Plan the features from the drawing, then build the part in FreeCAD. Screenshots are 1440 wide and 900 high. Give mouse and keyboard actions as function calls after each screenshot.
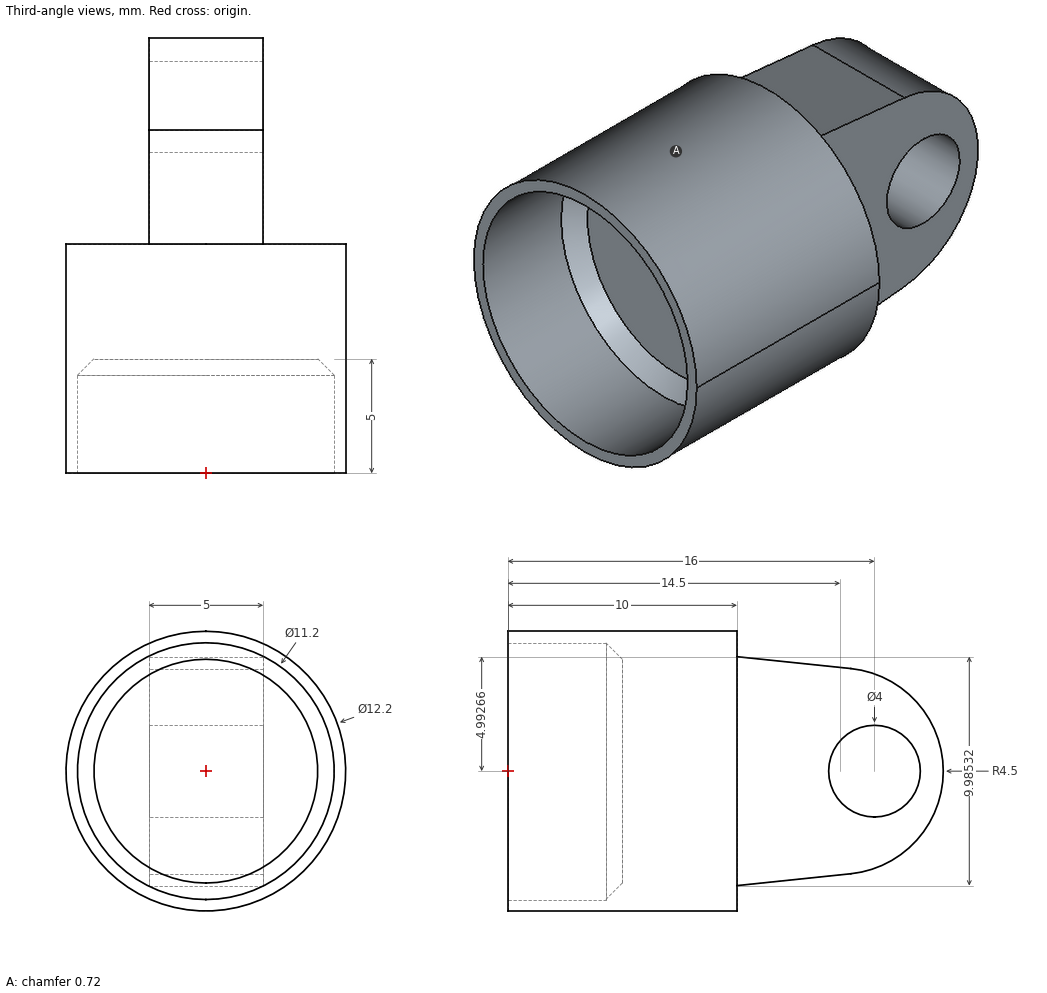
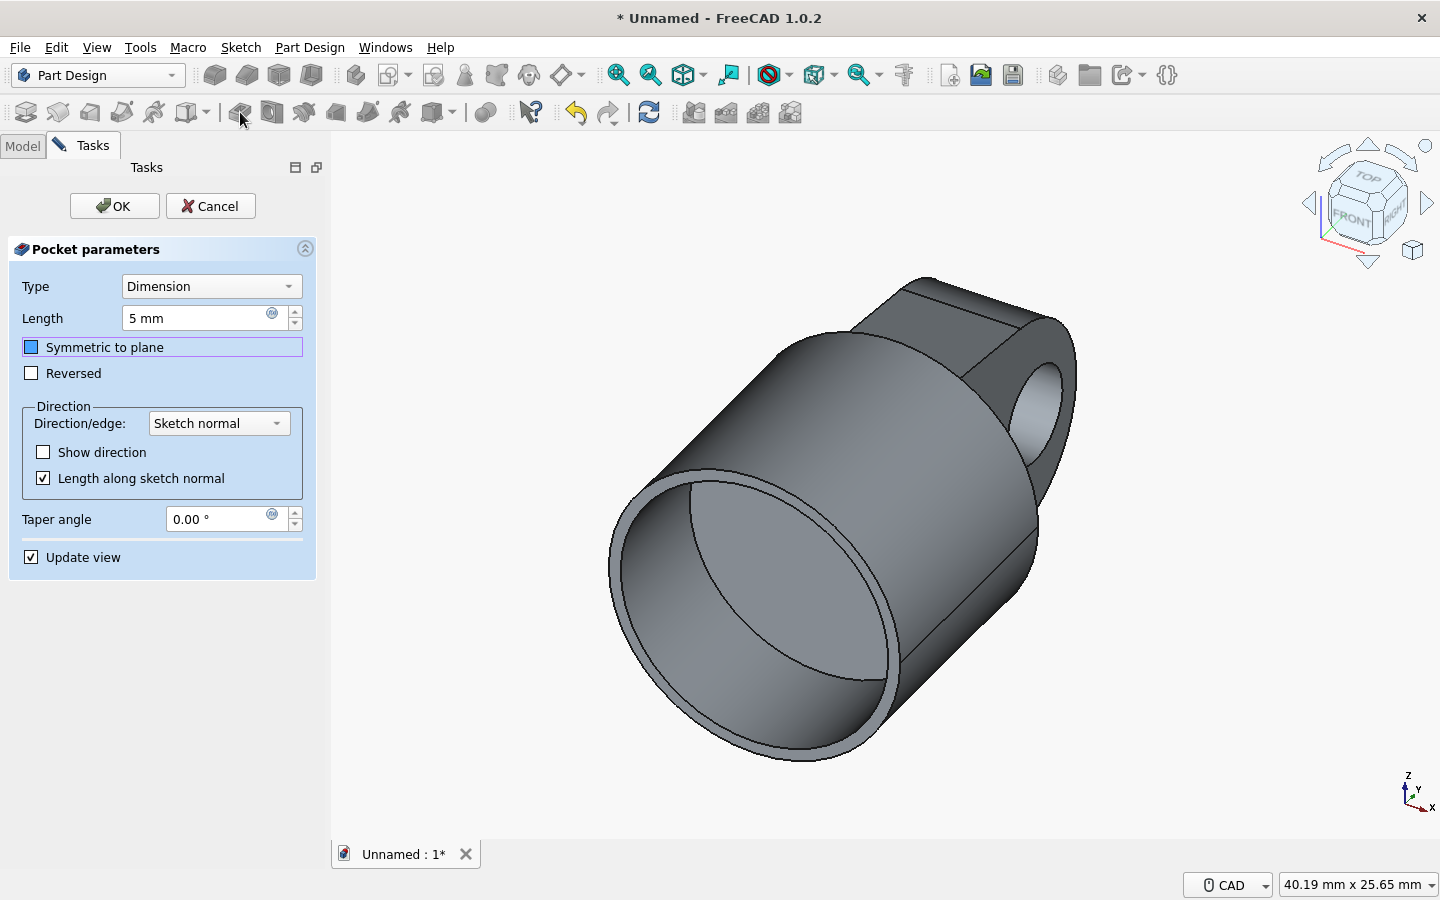
click(115, 206)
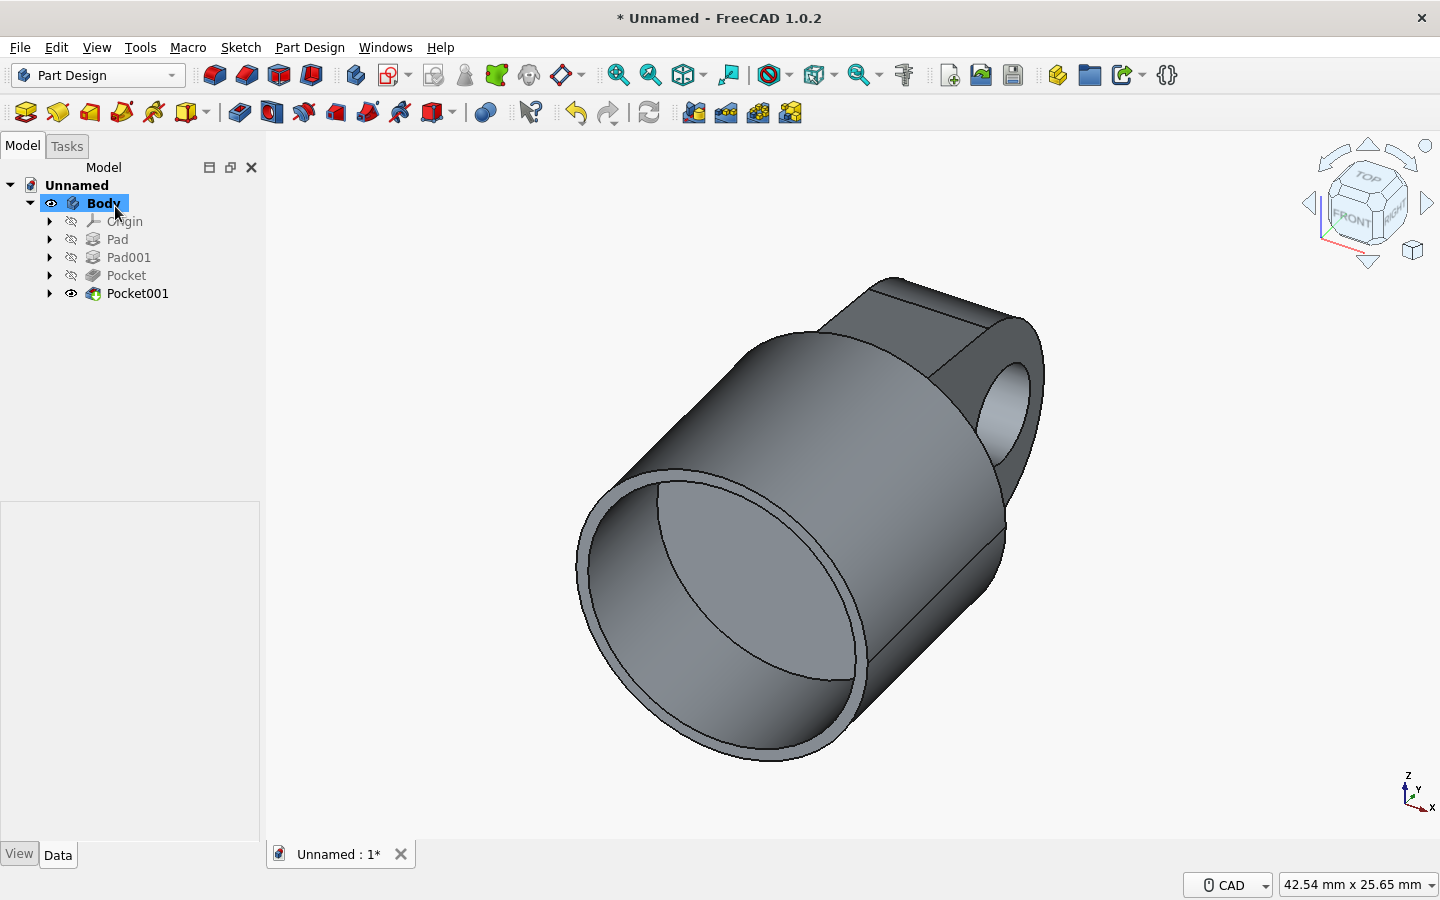
key(0)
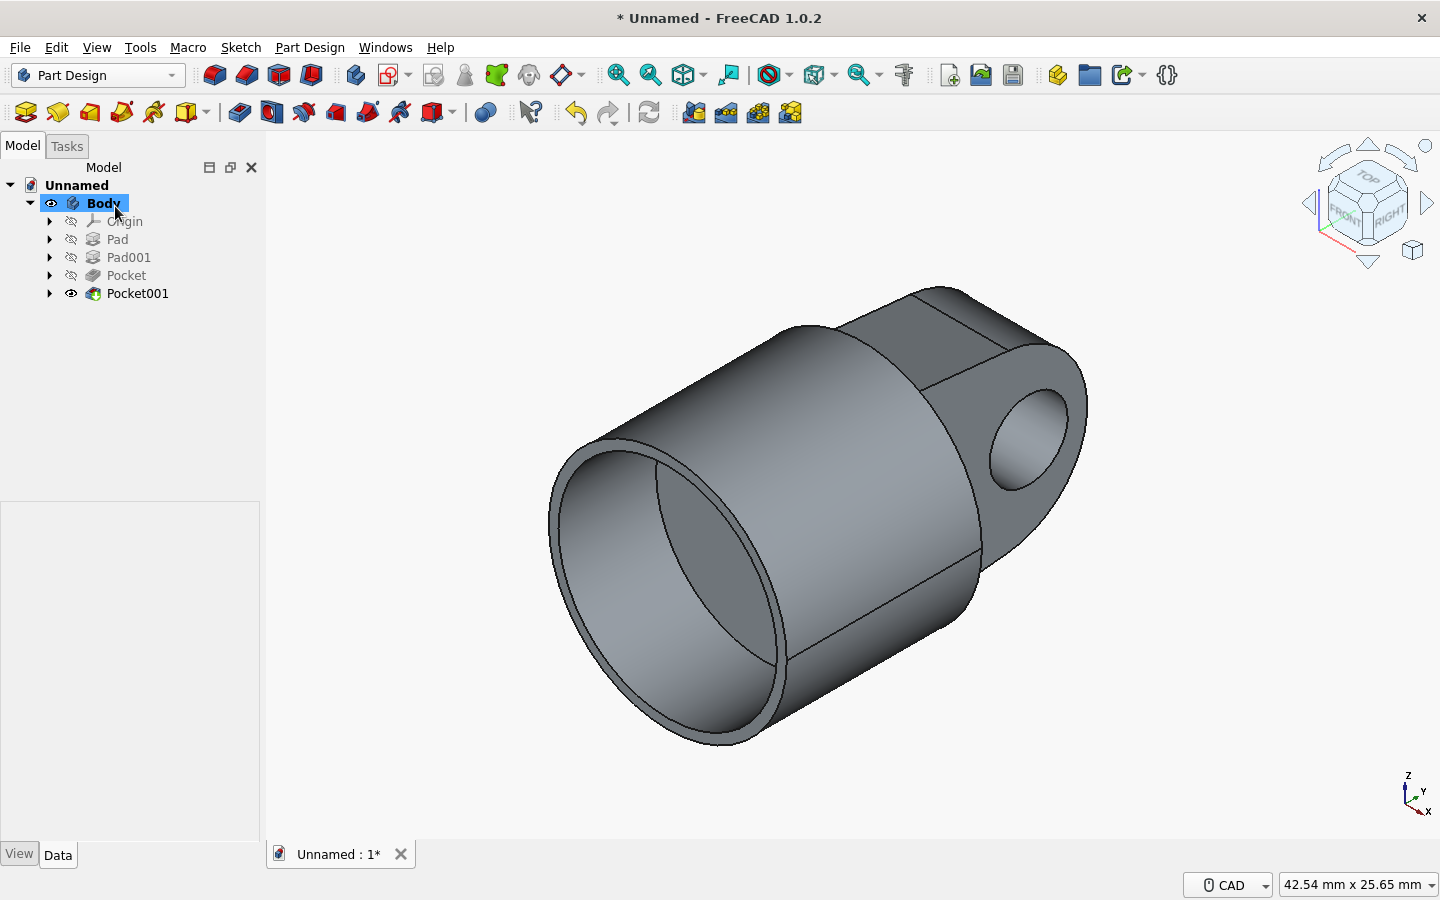
key(2)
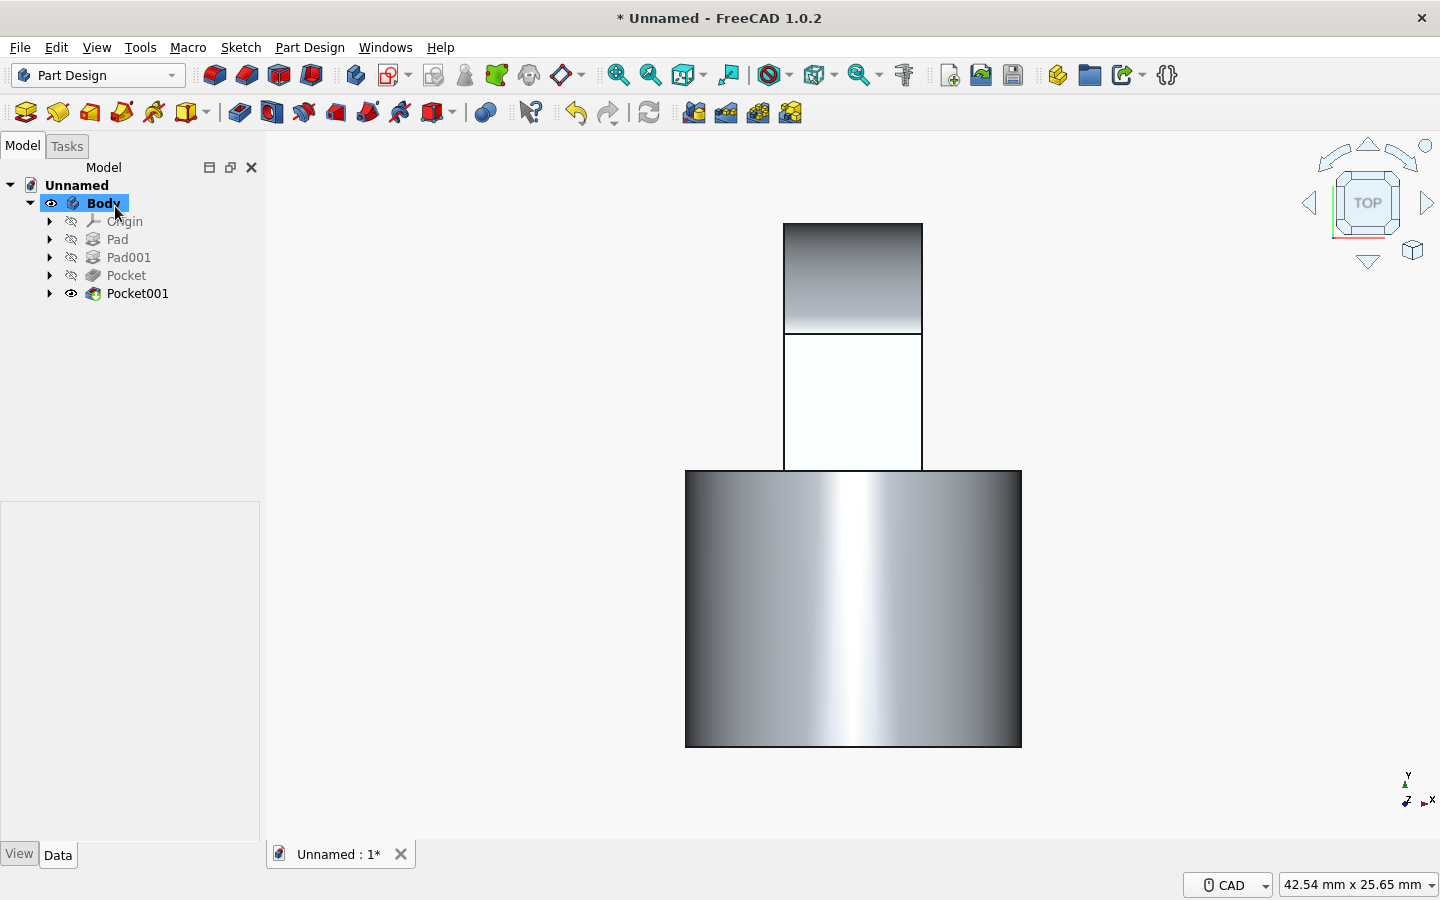
key(1)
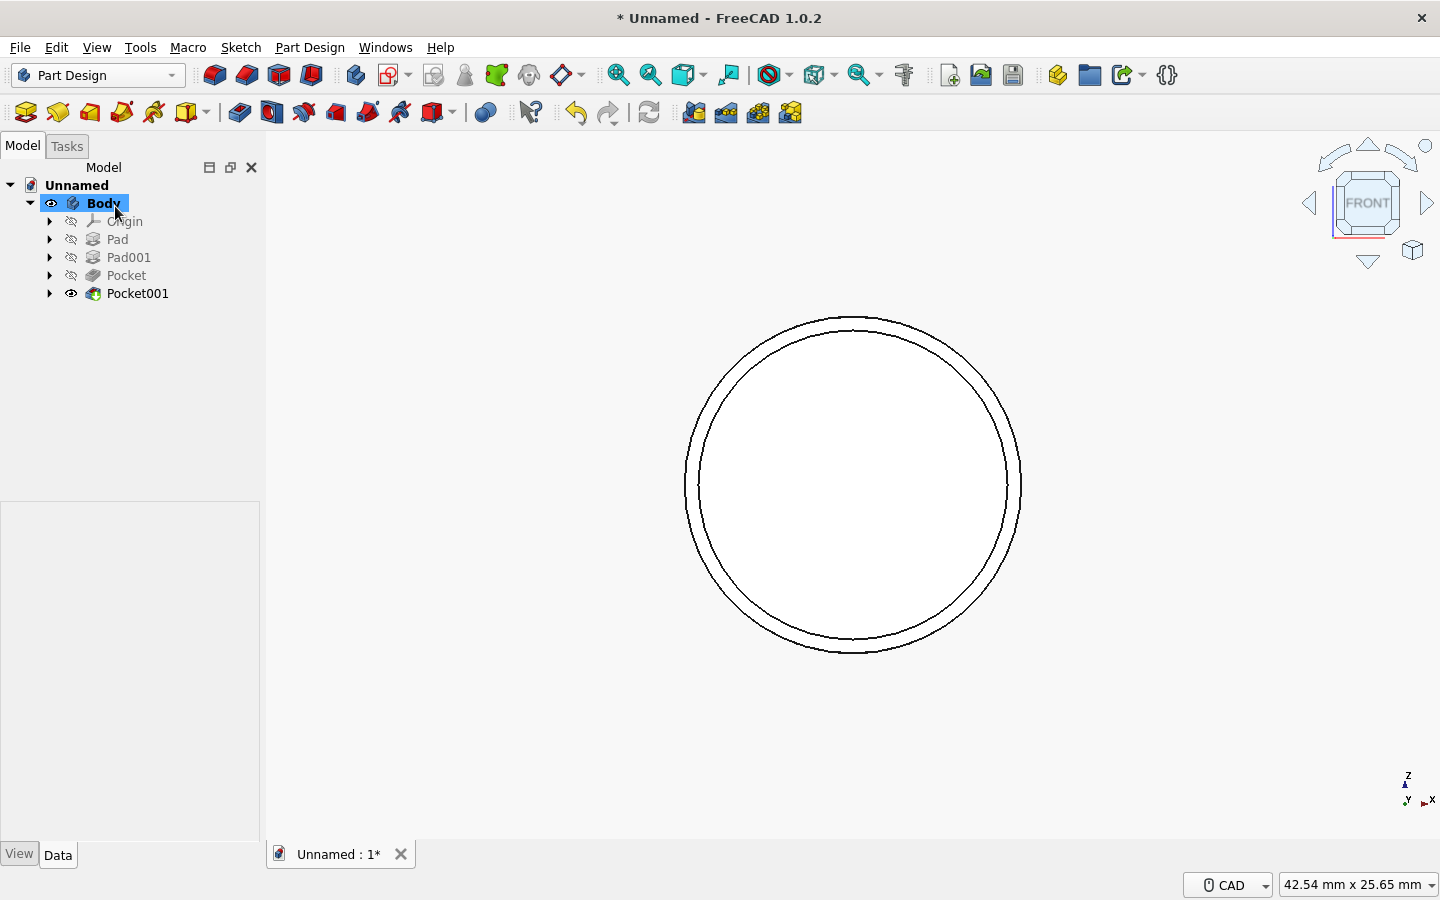
key(3)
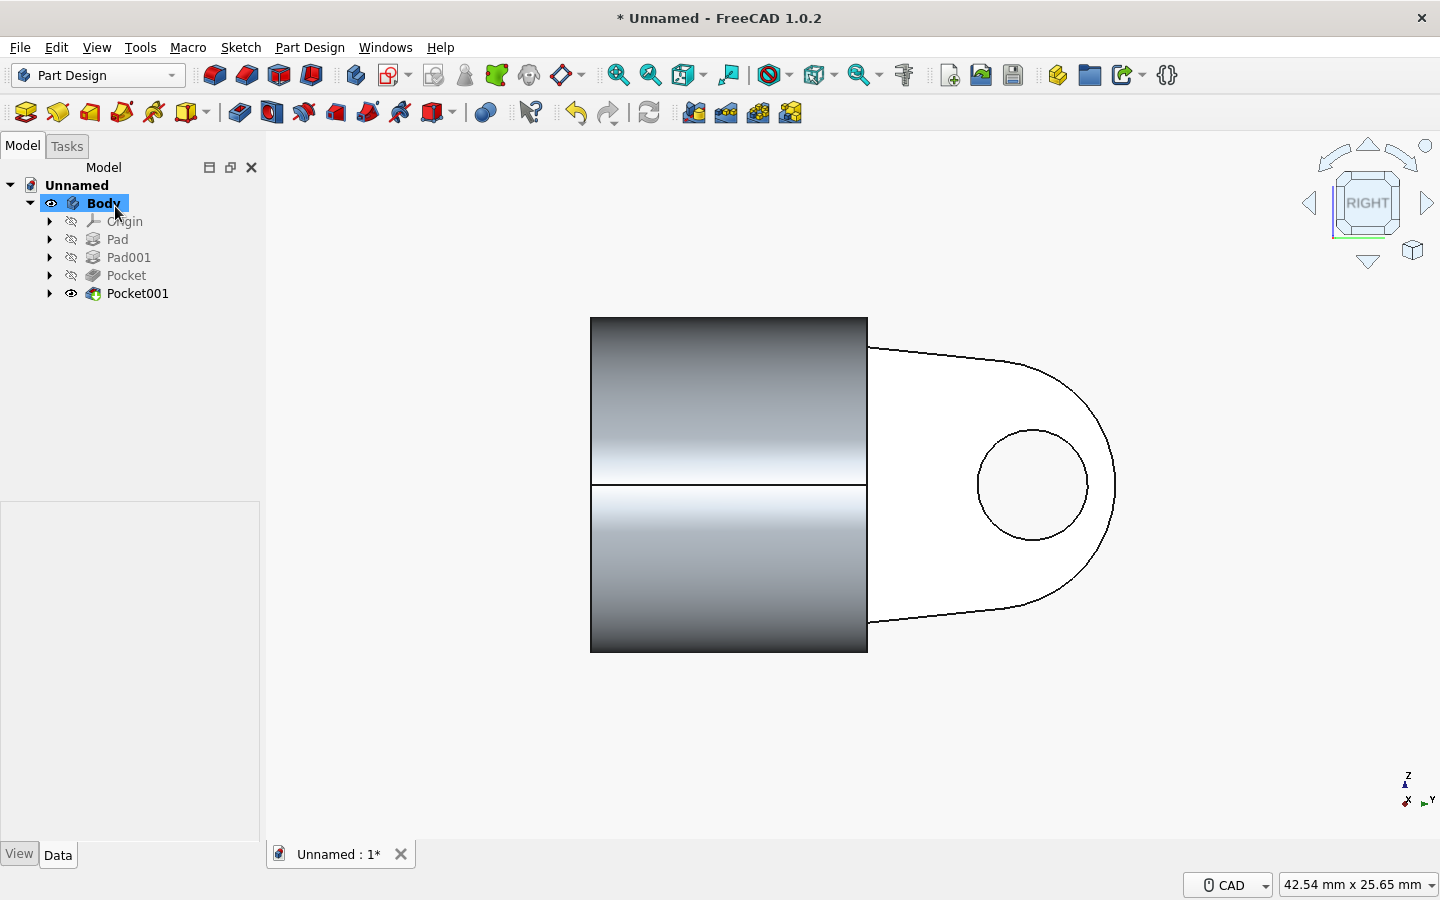
key(5)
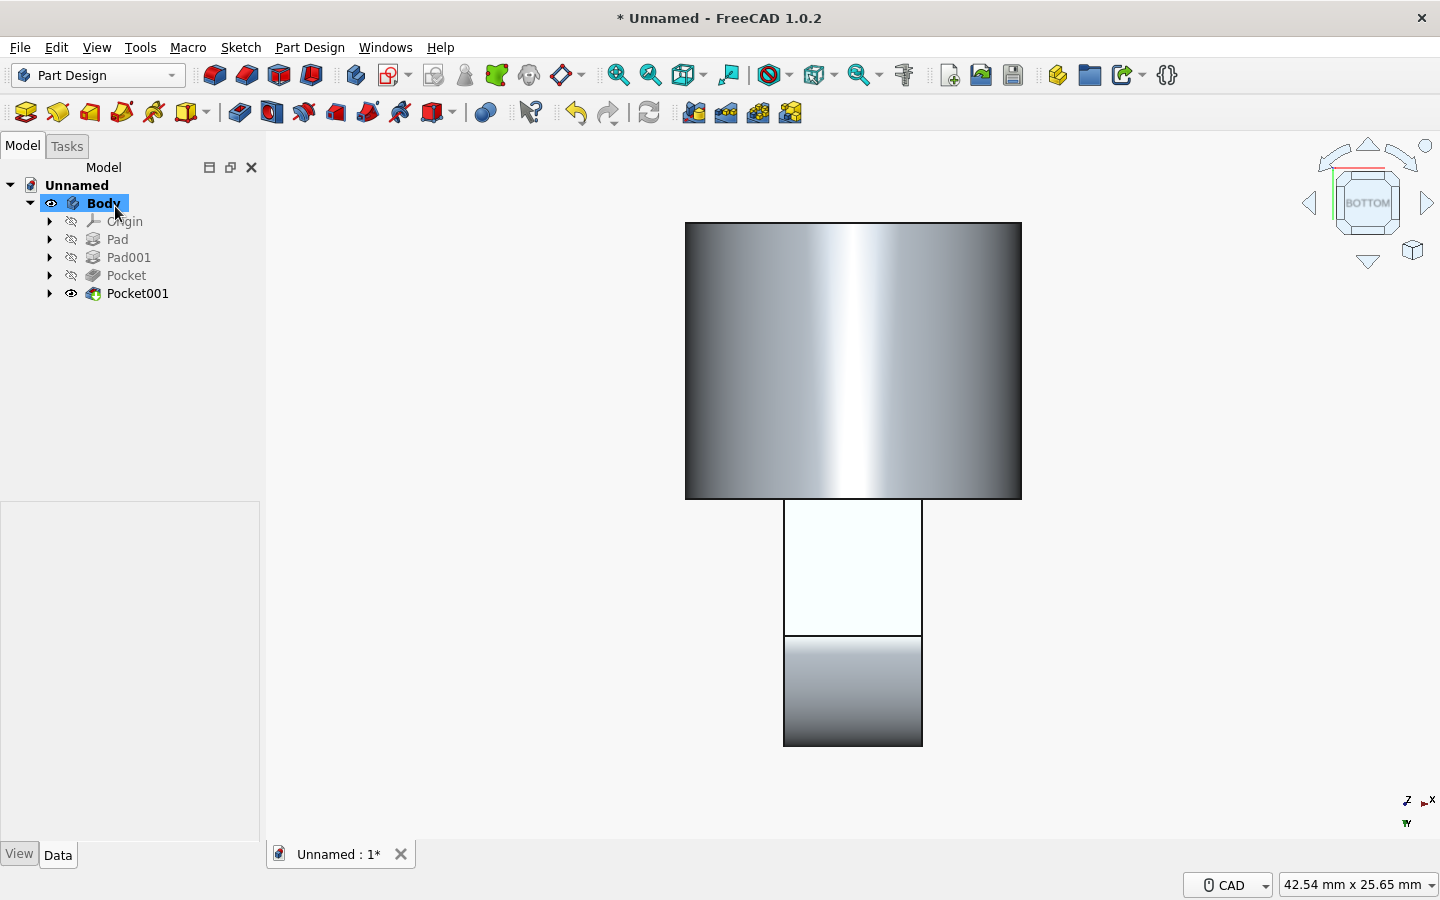
key(4)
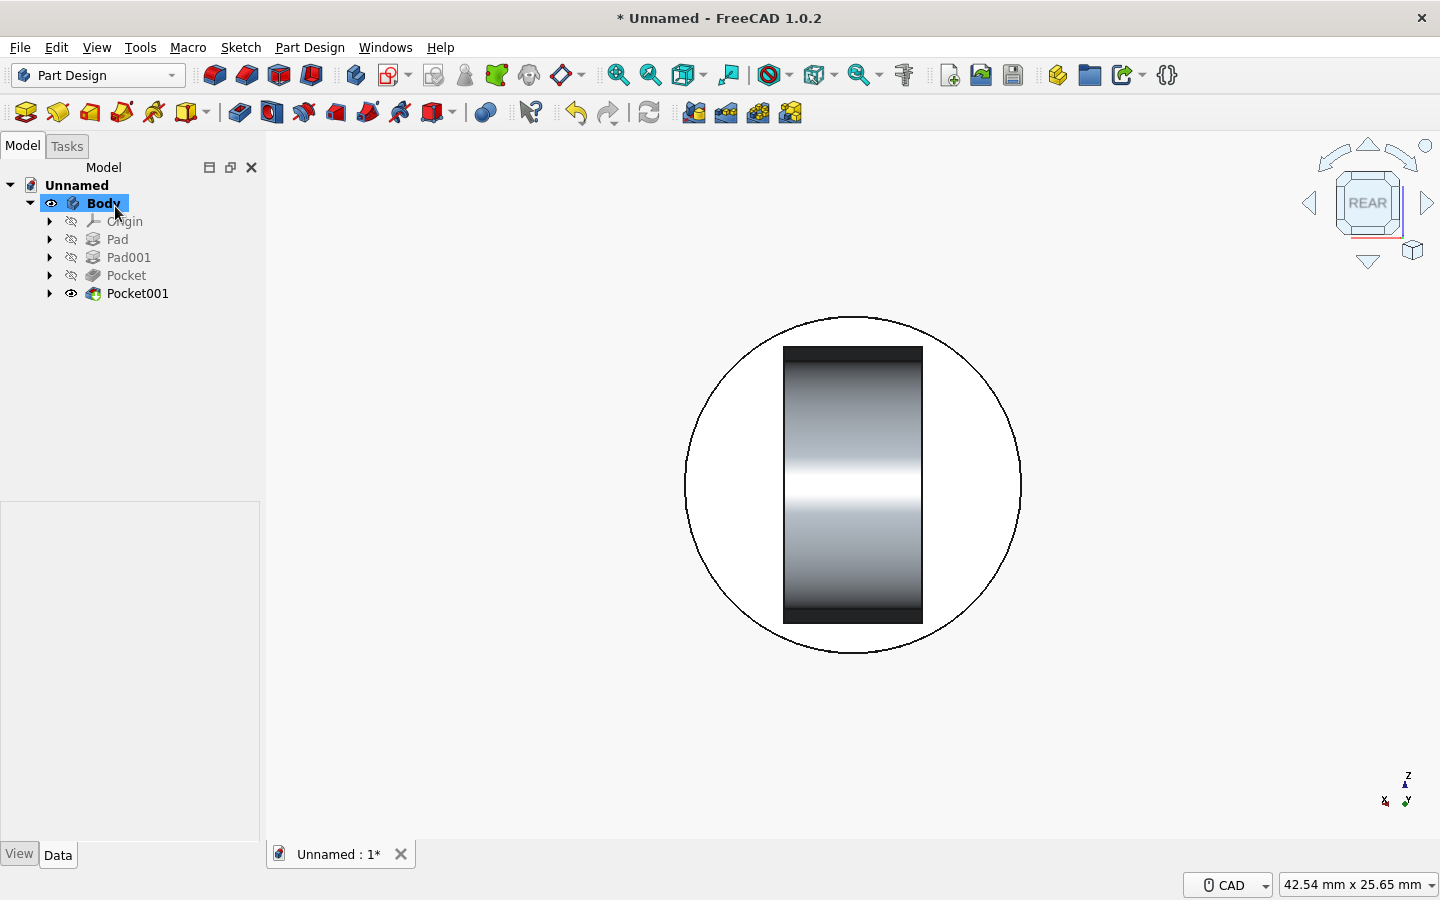
key(6)